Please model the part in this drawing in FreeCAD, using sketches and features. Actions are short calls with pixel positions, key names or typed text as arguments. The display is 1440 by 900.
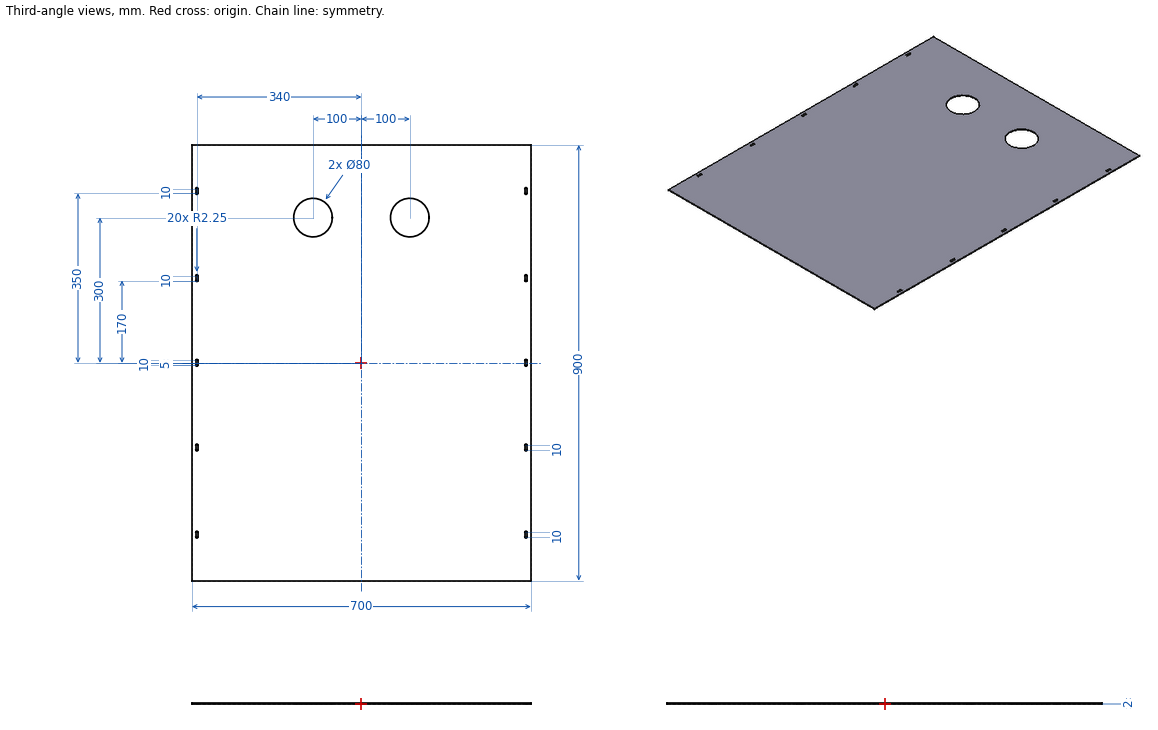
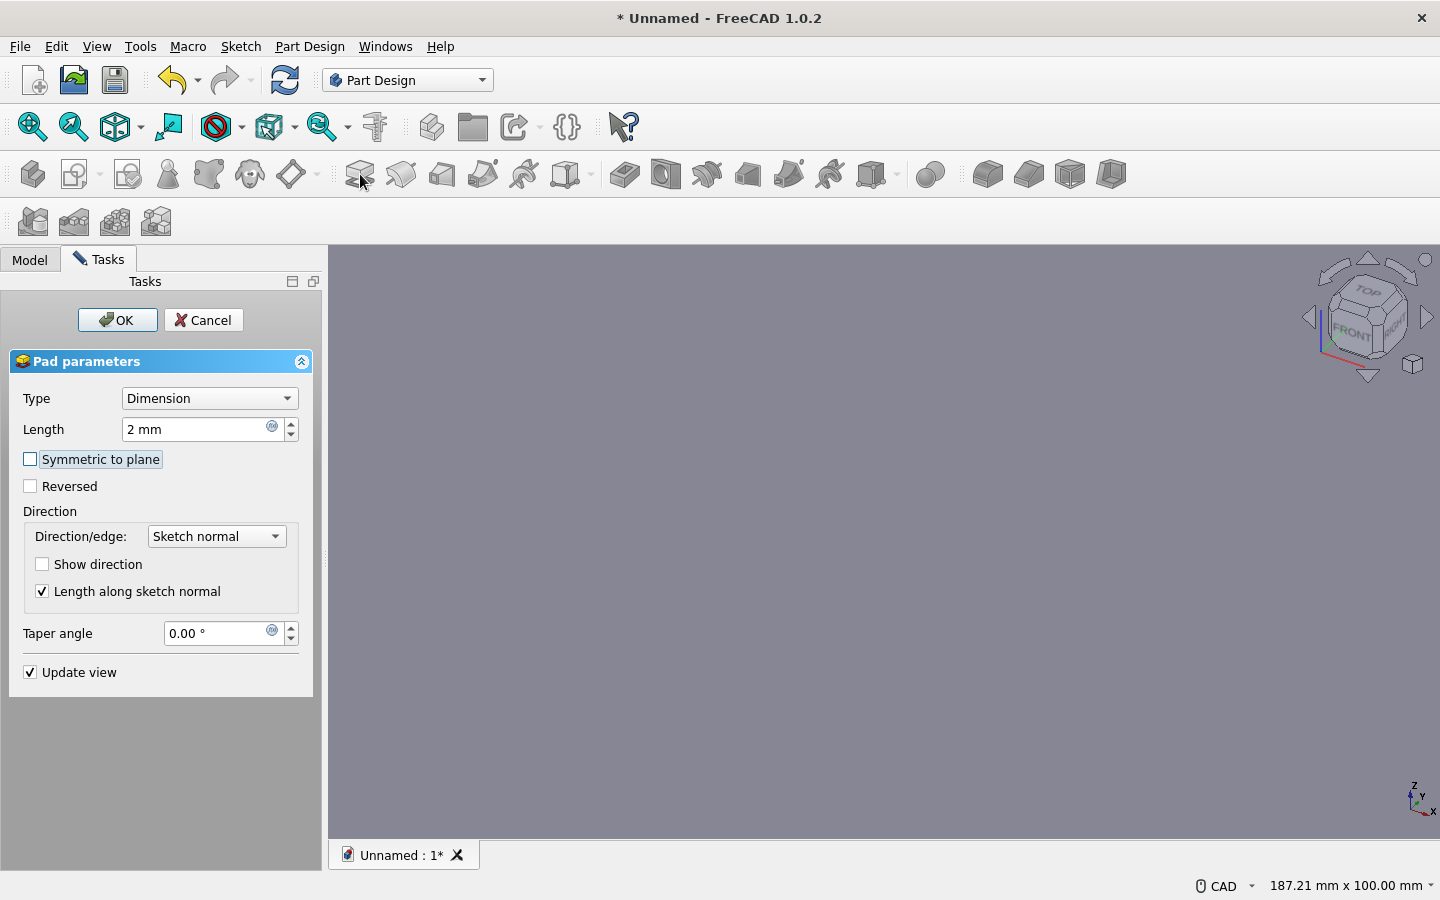
click(118, 320)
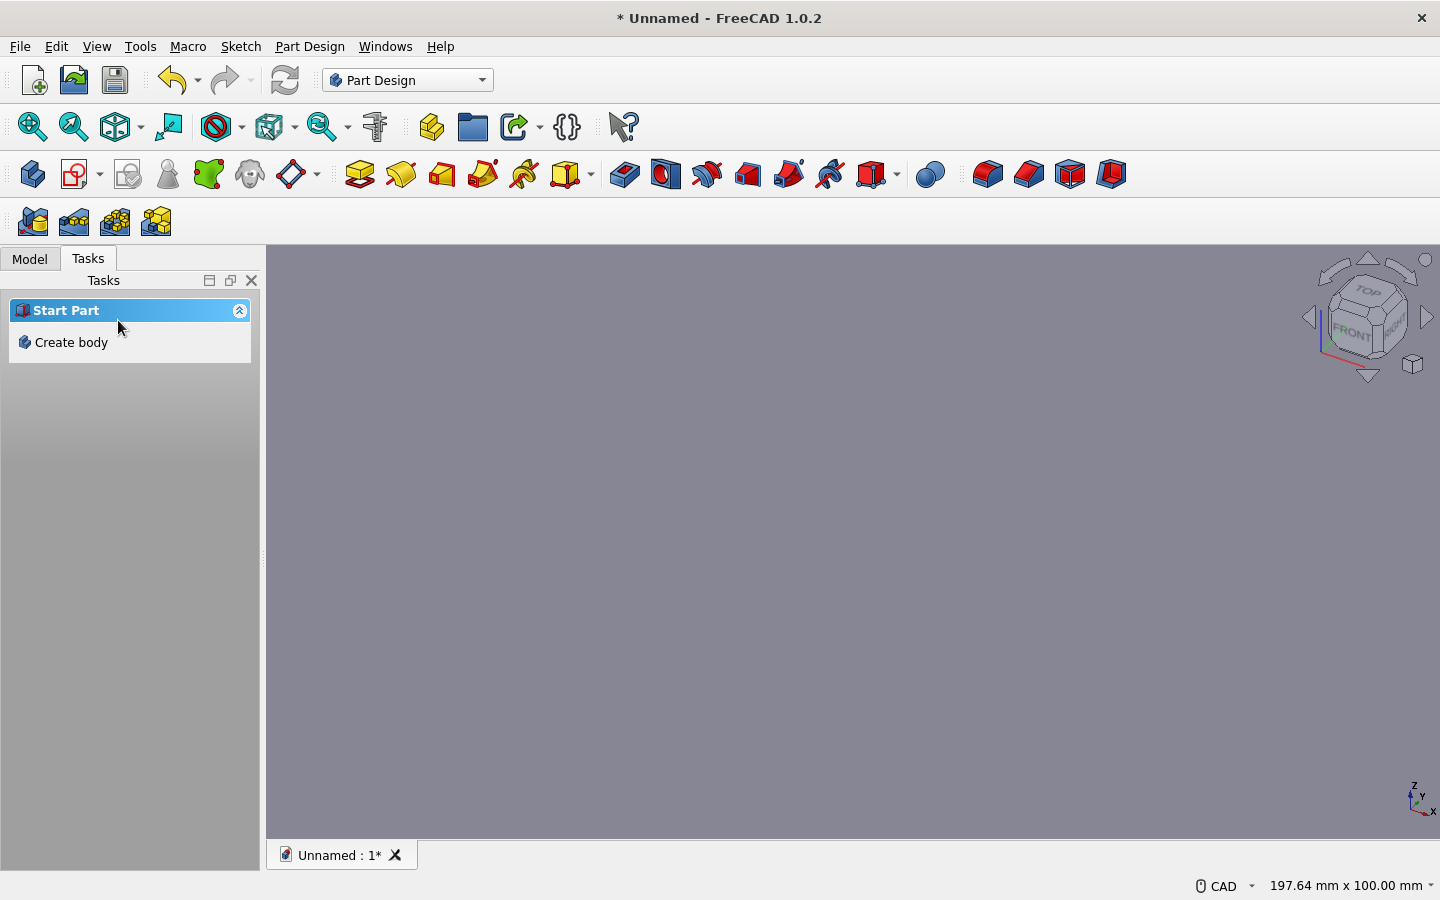
click(33, 128)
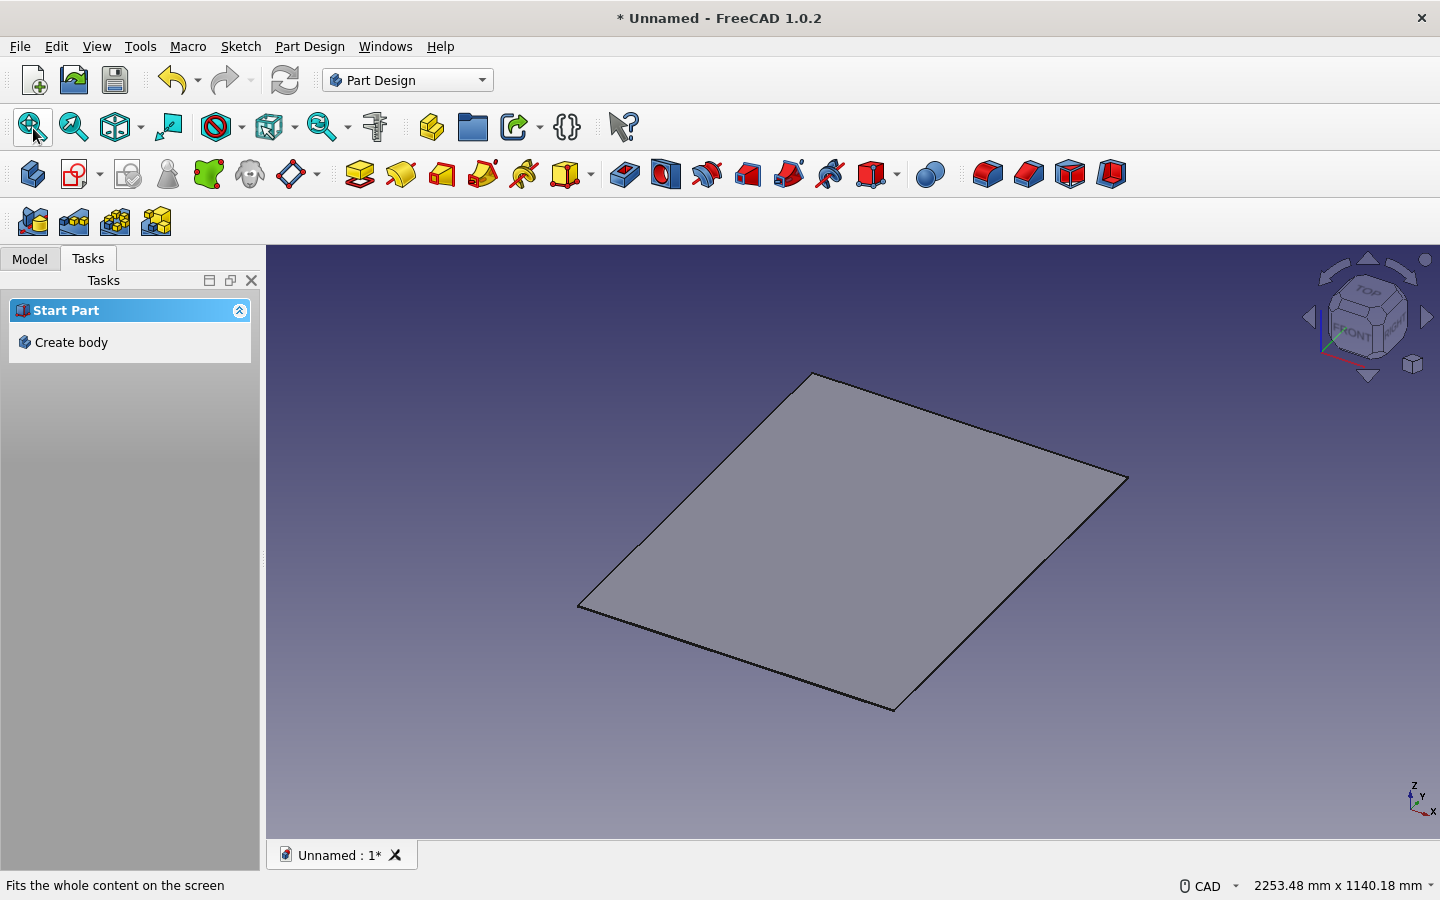
click(853, 541)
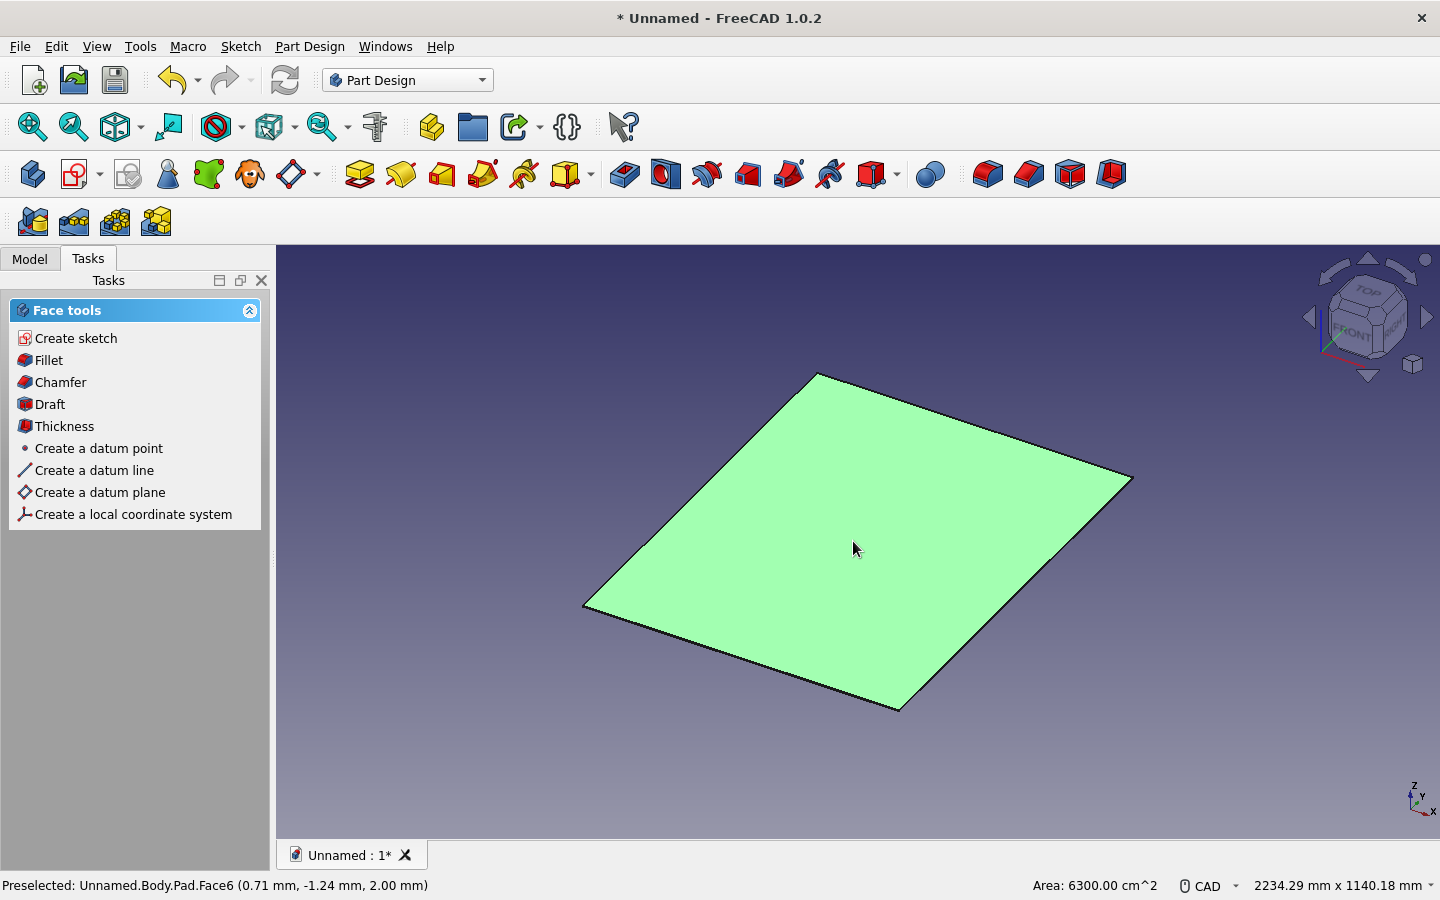
click(74, 174)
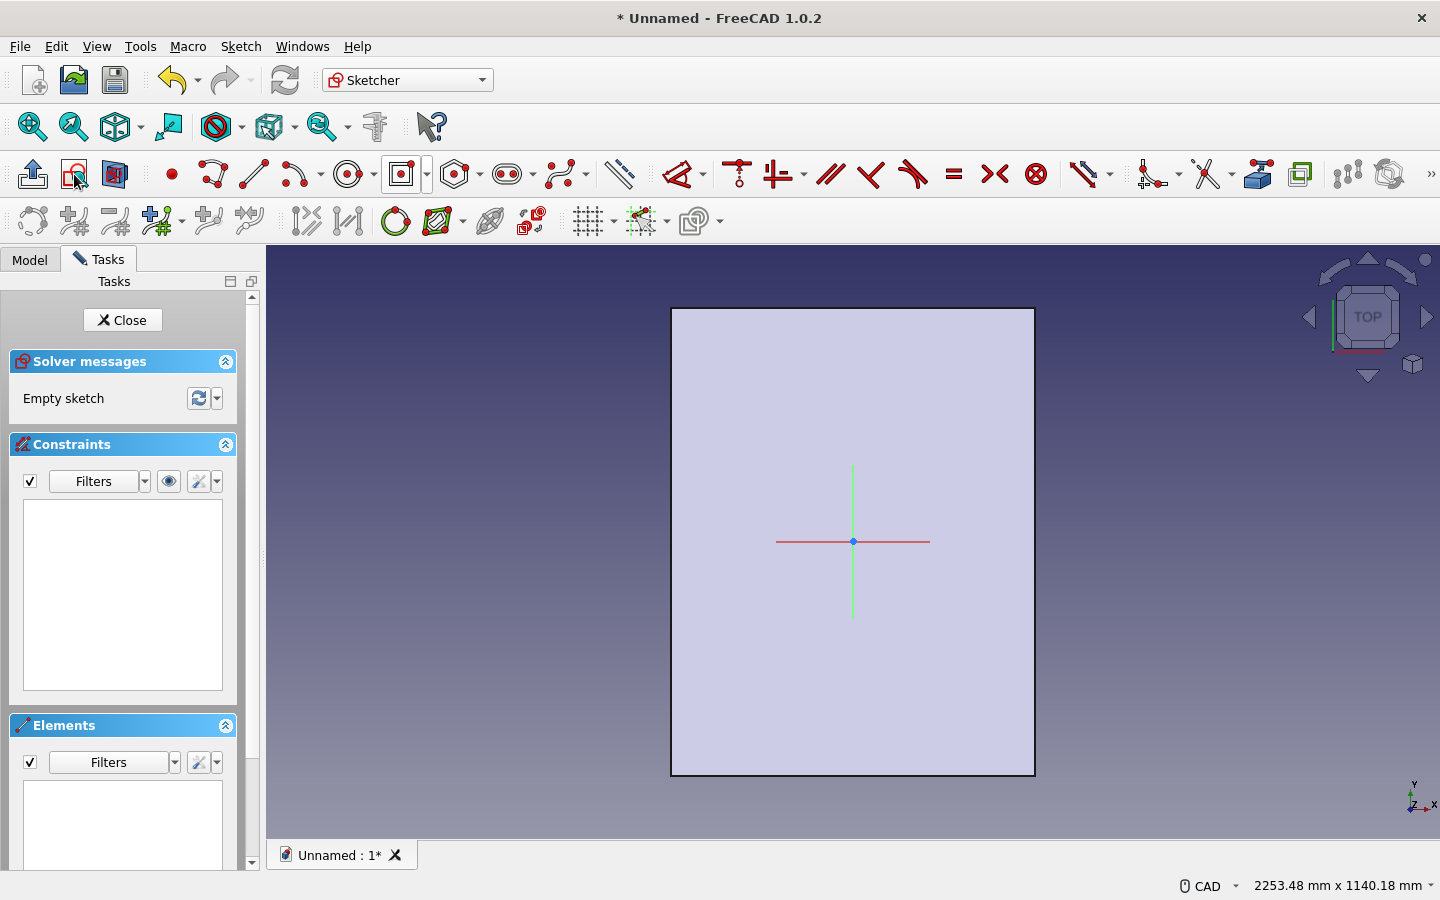
key(g)
key(s)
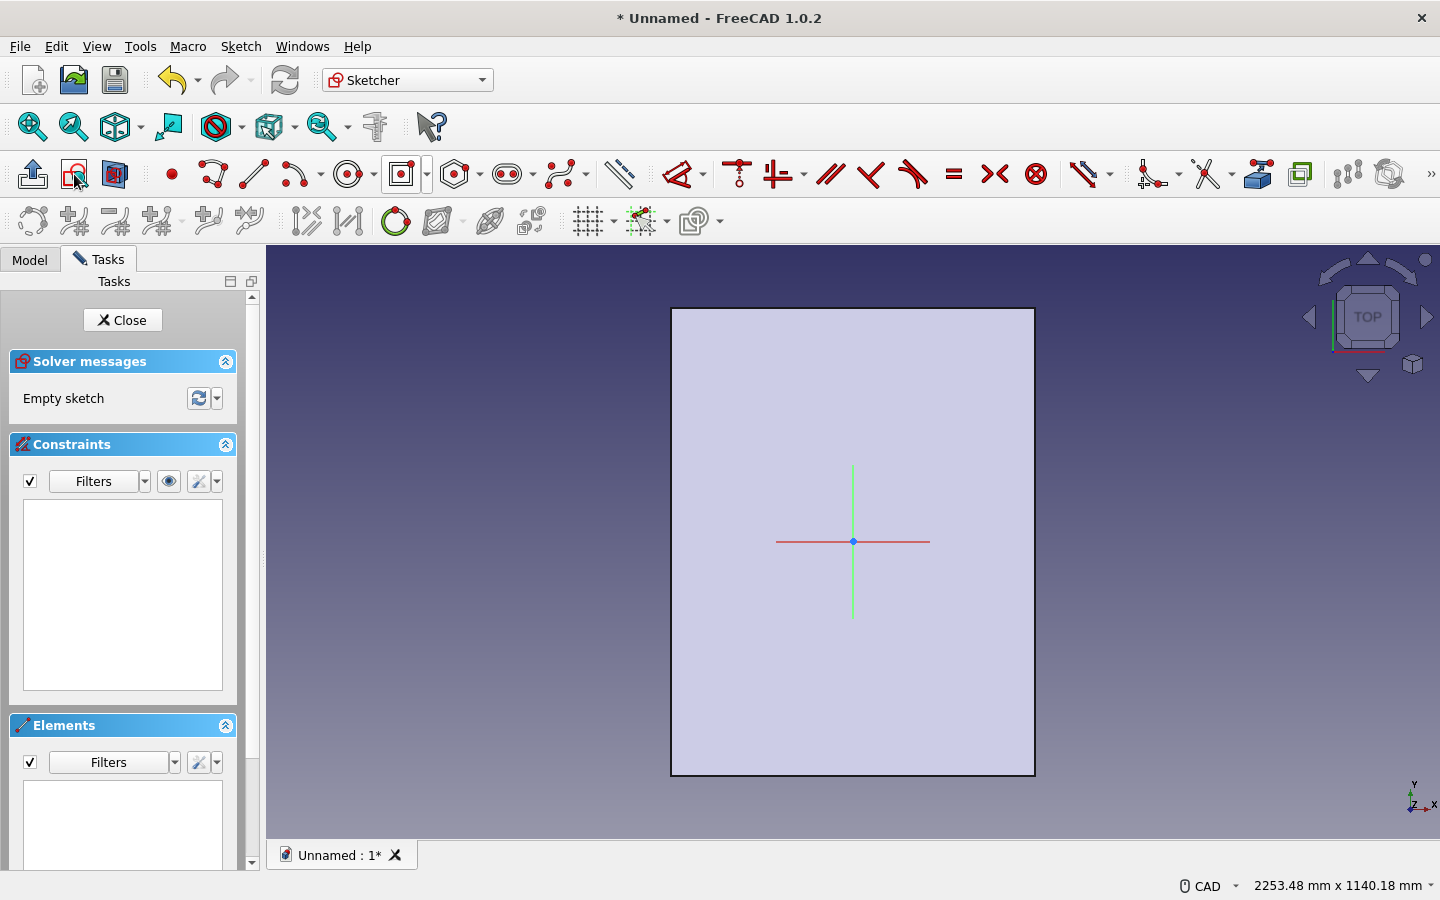
scroll(676, 453, up, 15)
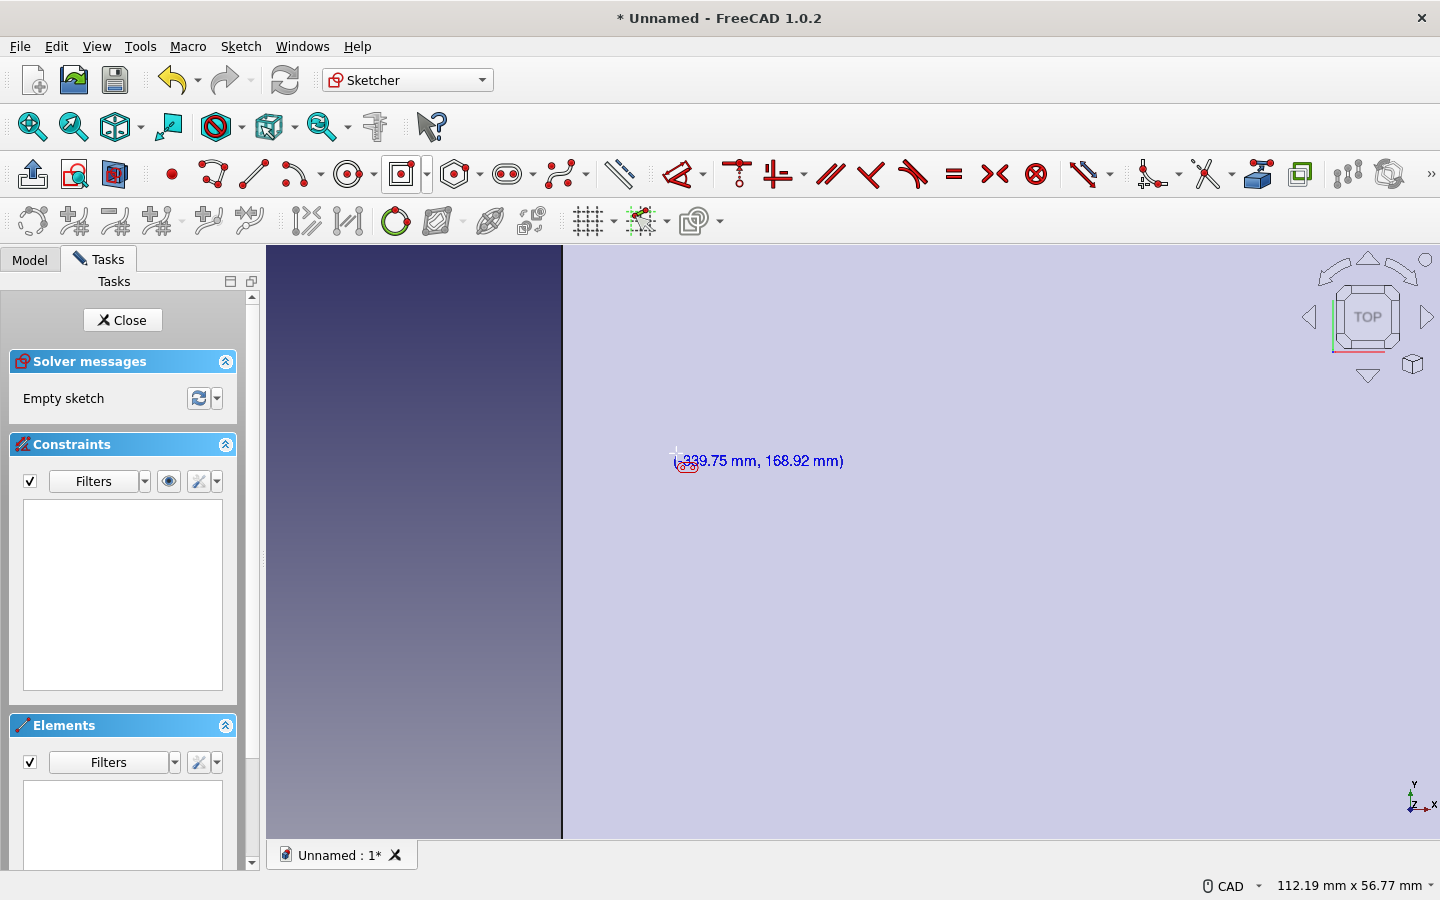
scroll(604, 453, down, 15)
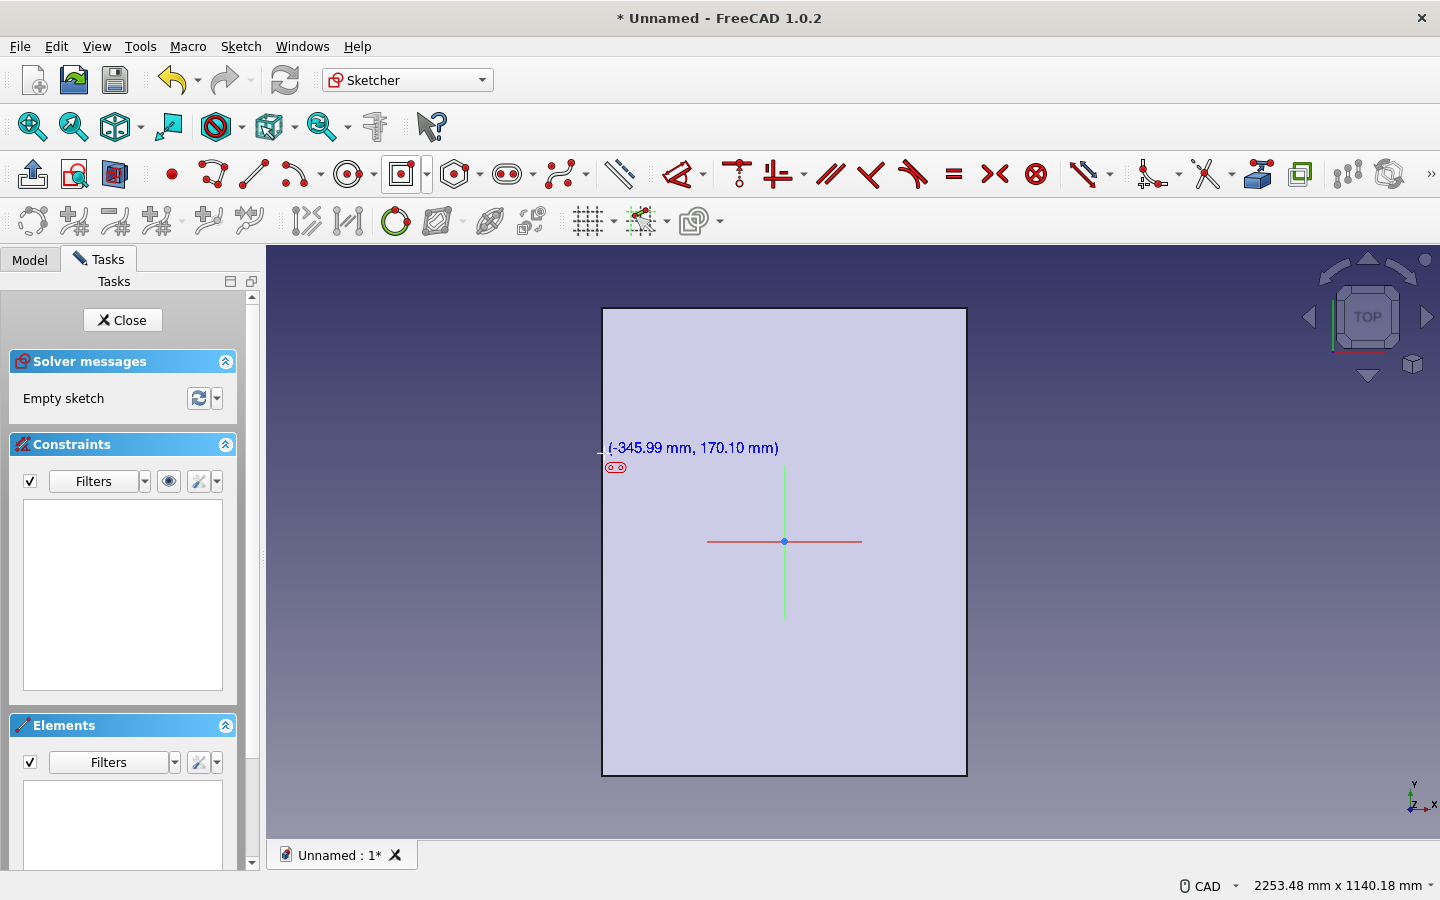
click(607, 453)